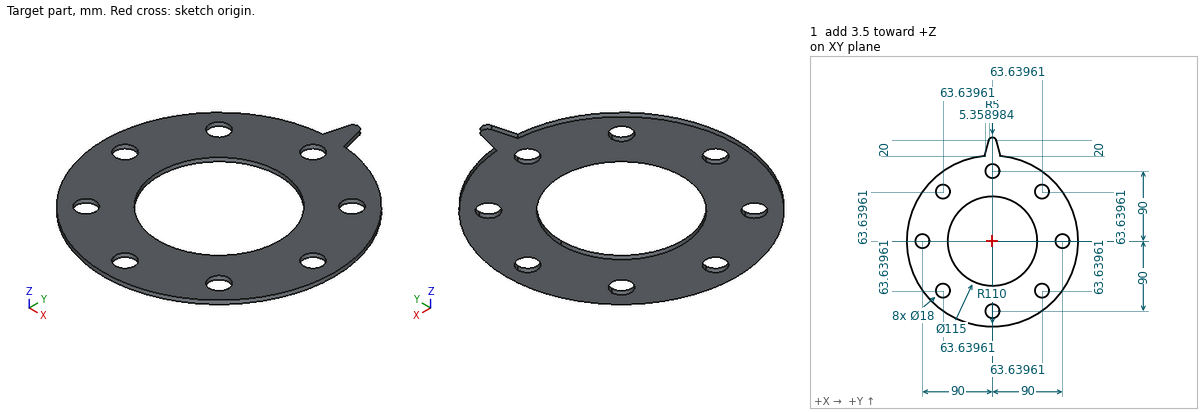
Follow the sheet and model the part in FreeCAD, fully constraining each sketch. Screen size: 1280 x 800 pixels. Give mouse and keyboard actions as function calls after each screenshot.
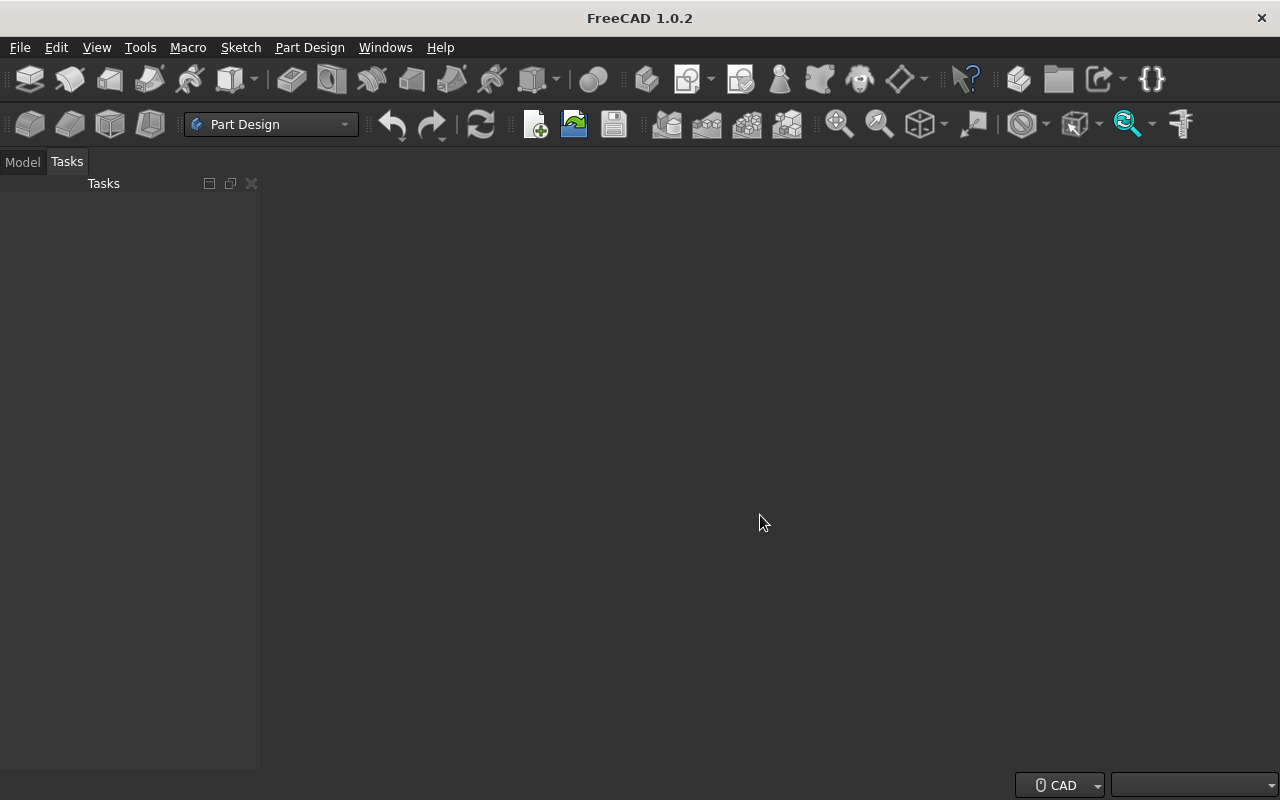
click(534, 124)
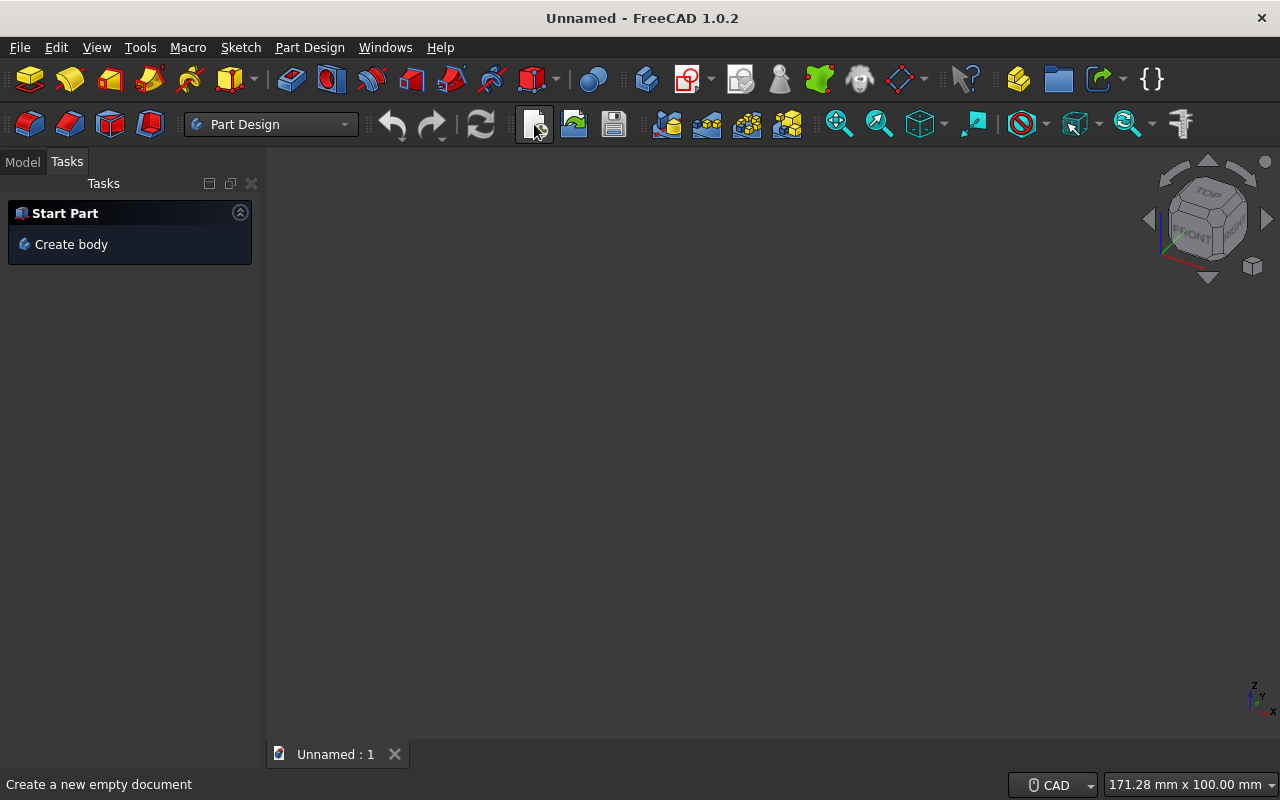
click(688, 80)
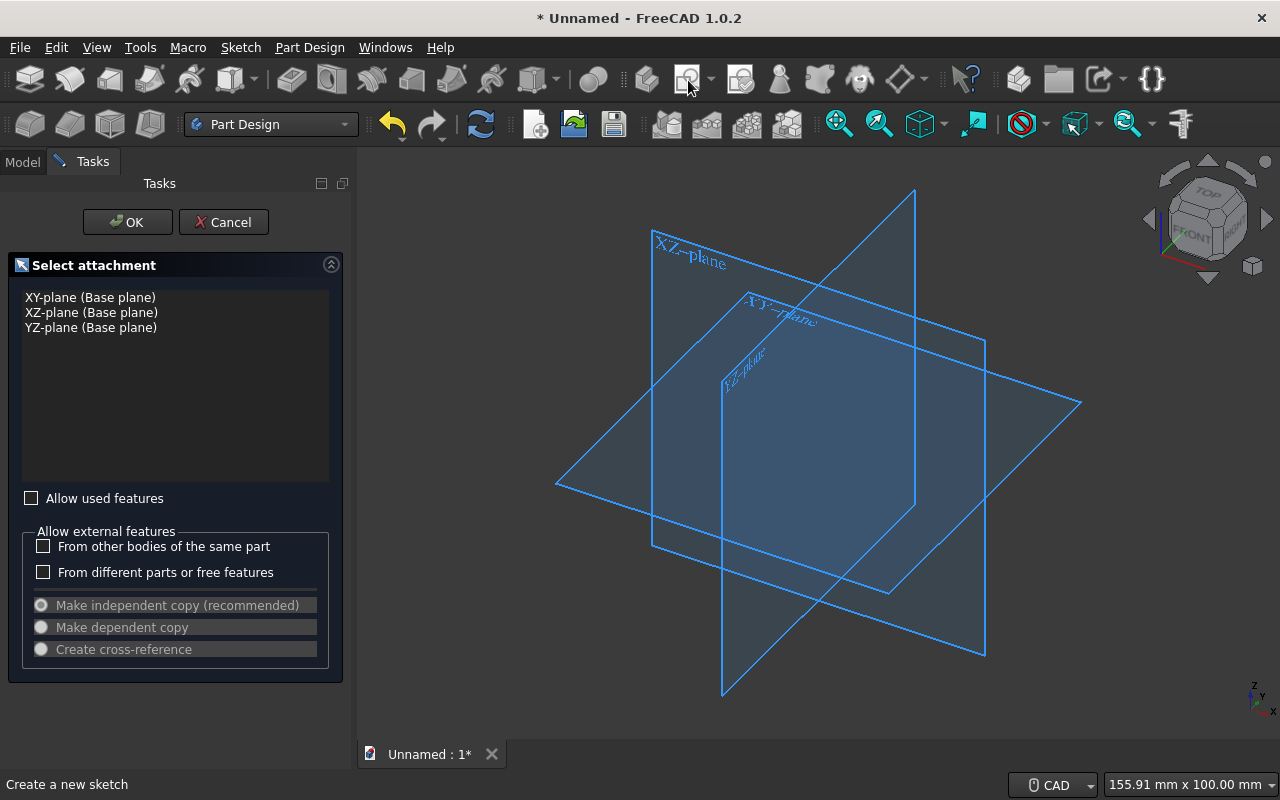
click(82, 298)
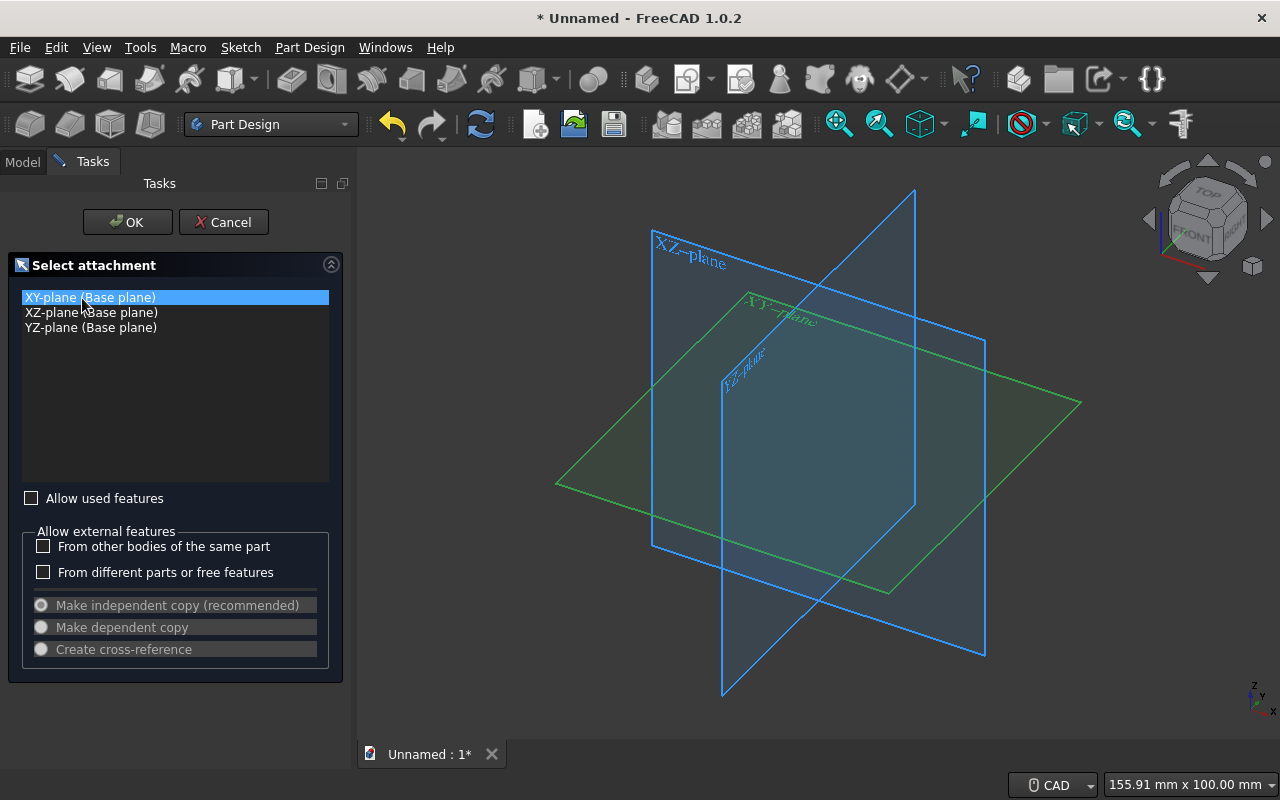
click(128, 222)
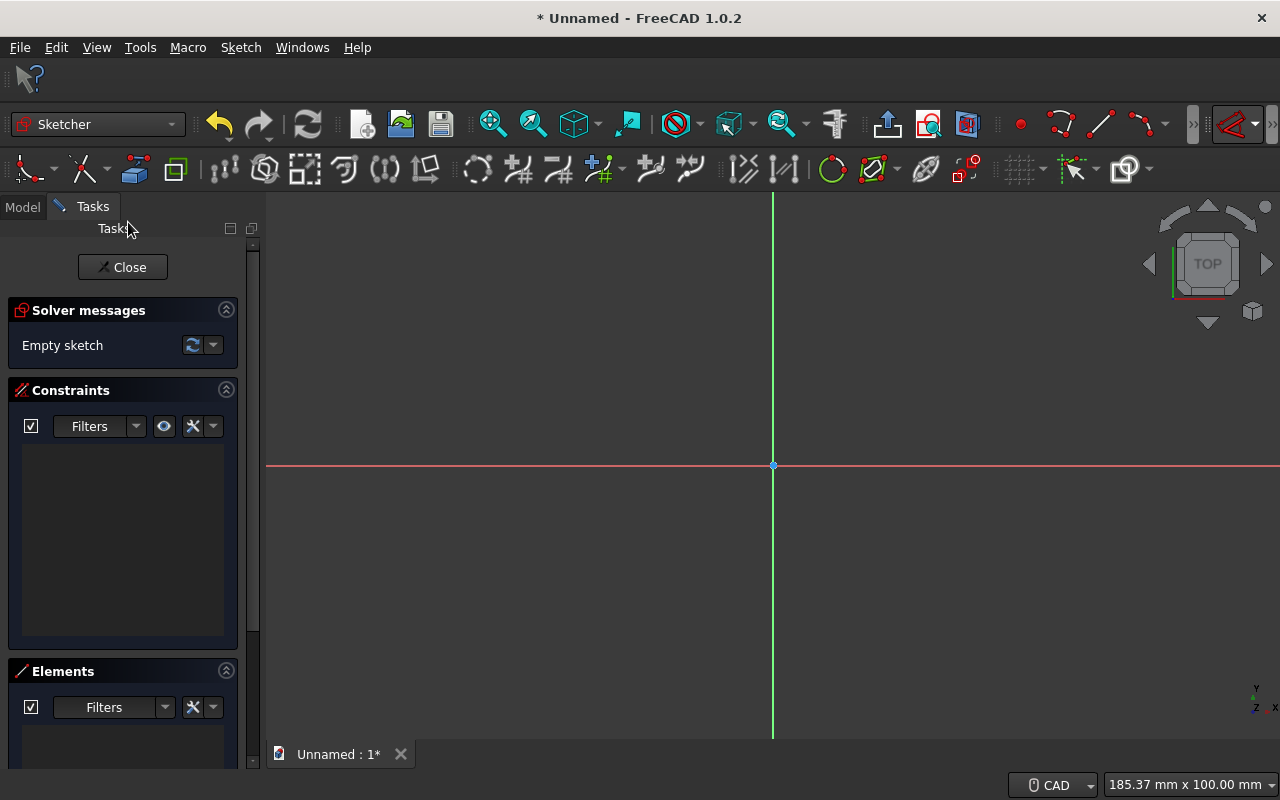
scroll(682, 486, down, 7)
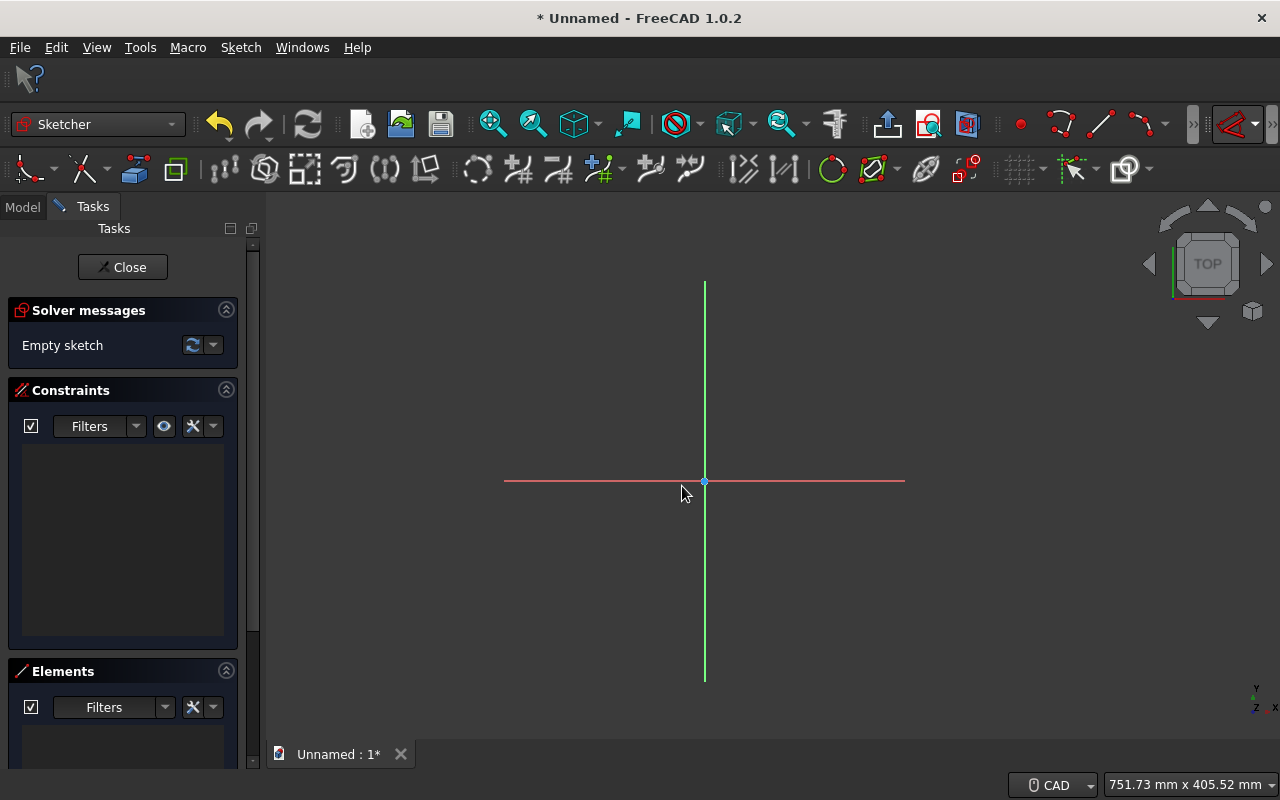
click(1102, 124)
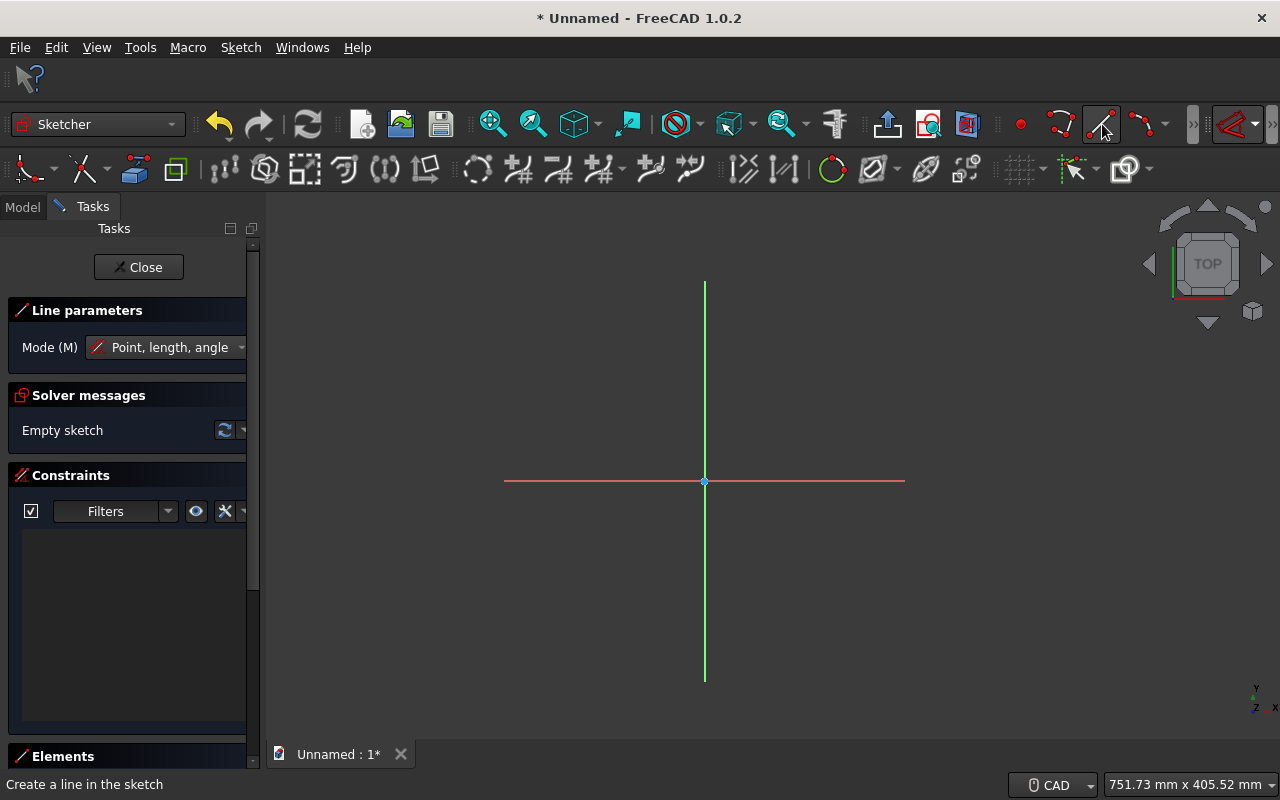
scroll(698, 307, up, 5)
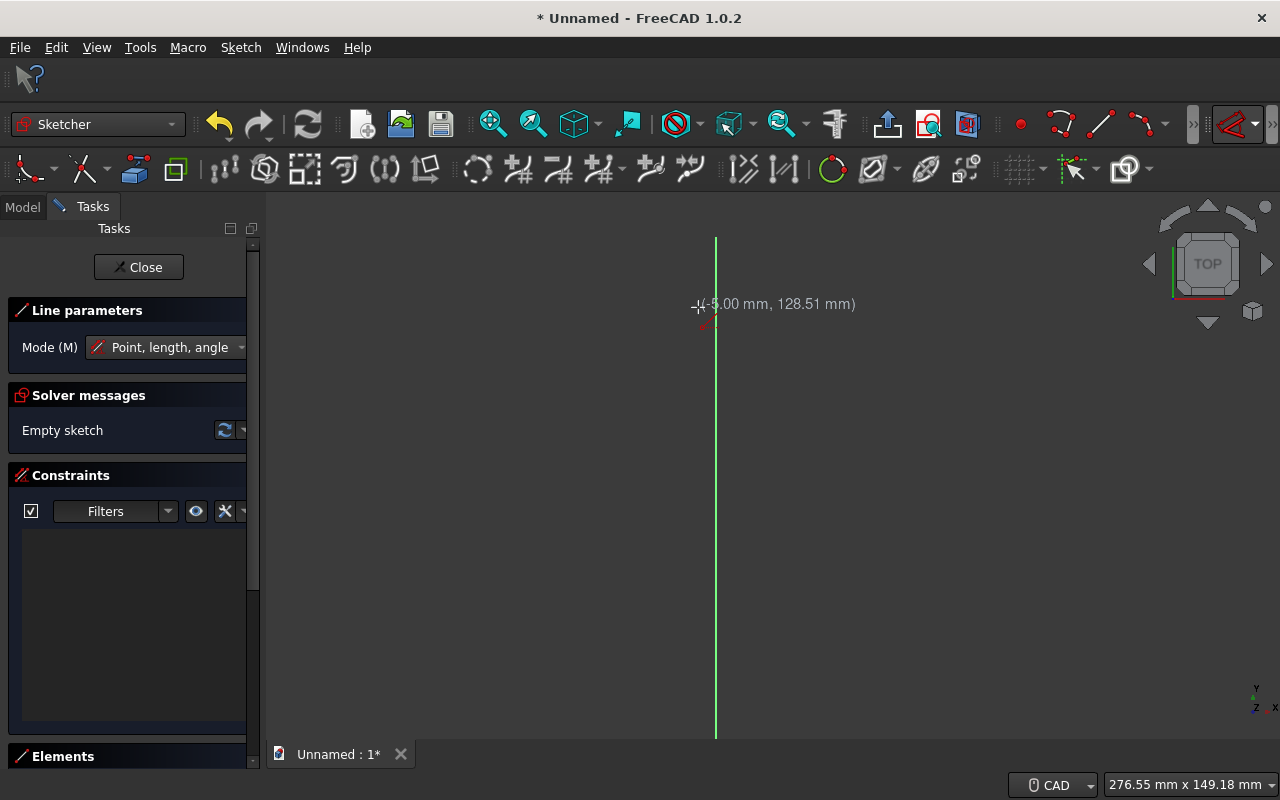
click(698, 306)
click(678, 379)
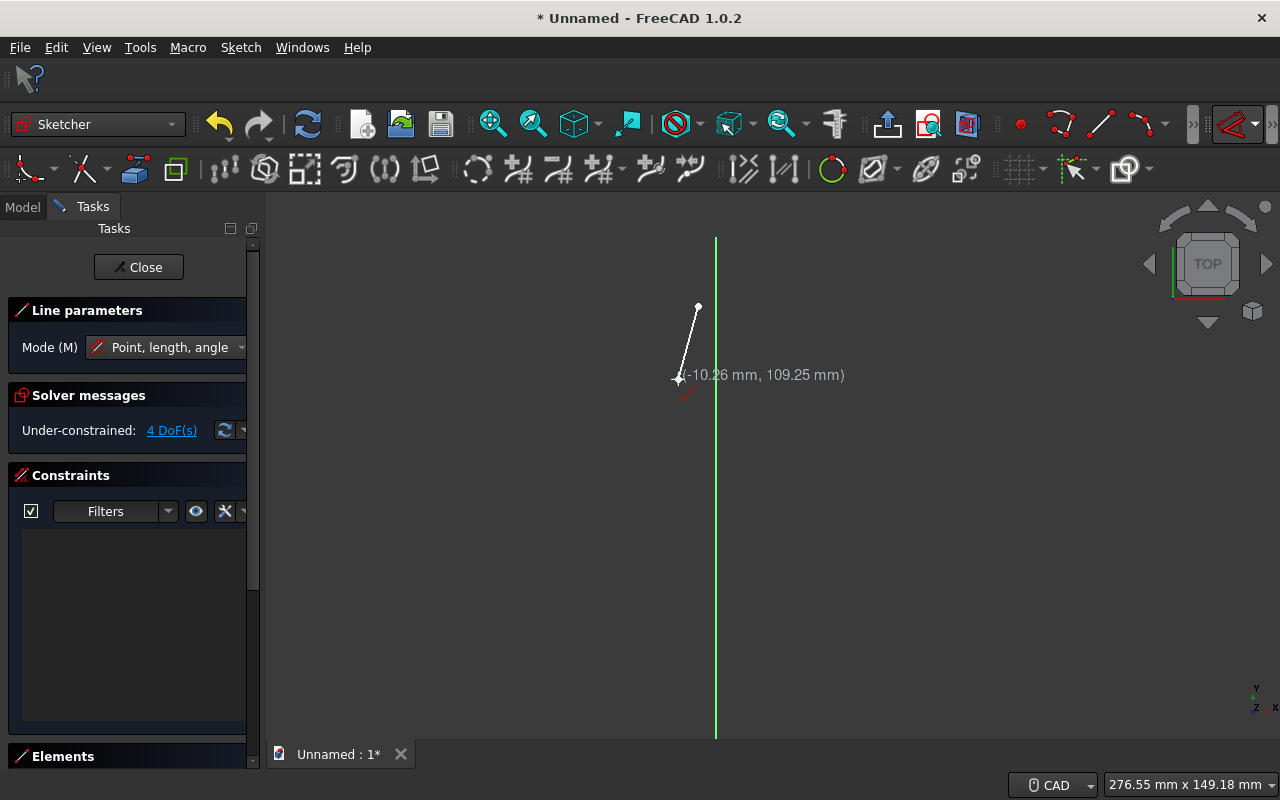
click(753, 379)
click(733, 306)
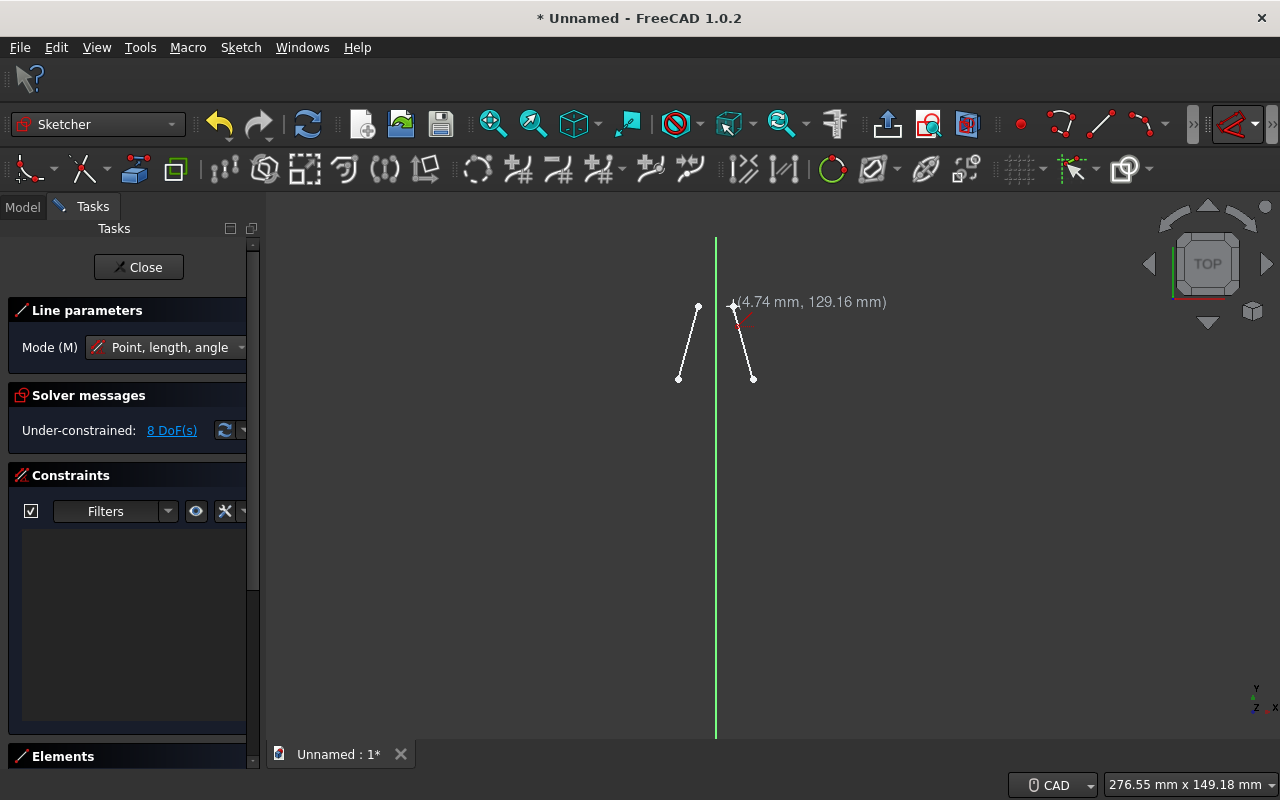
click(1142, 124)